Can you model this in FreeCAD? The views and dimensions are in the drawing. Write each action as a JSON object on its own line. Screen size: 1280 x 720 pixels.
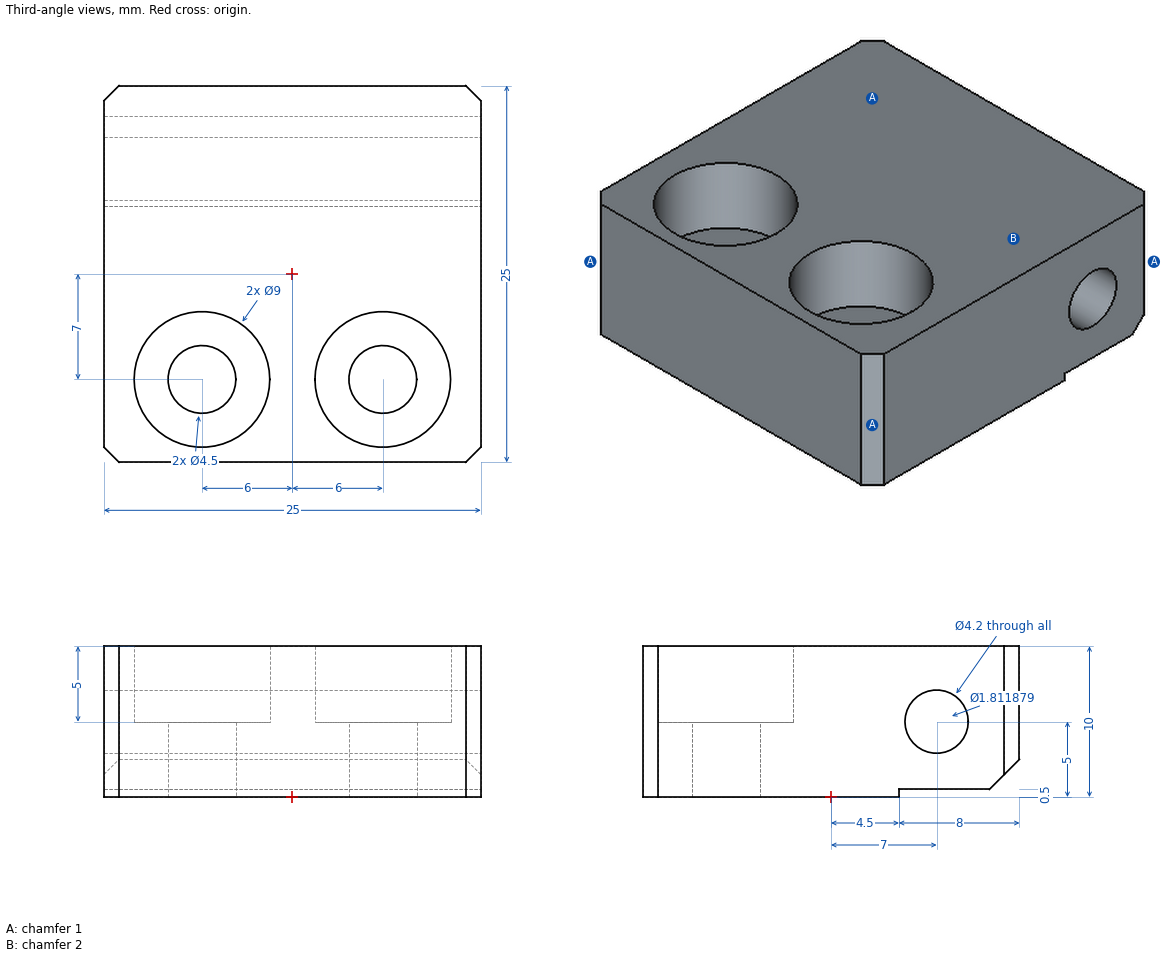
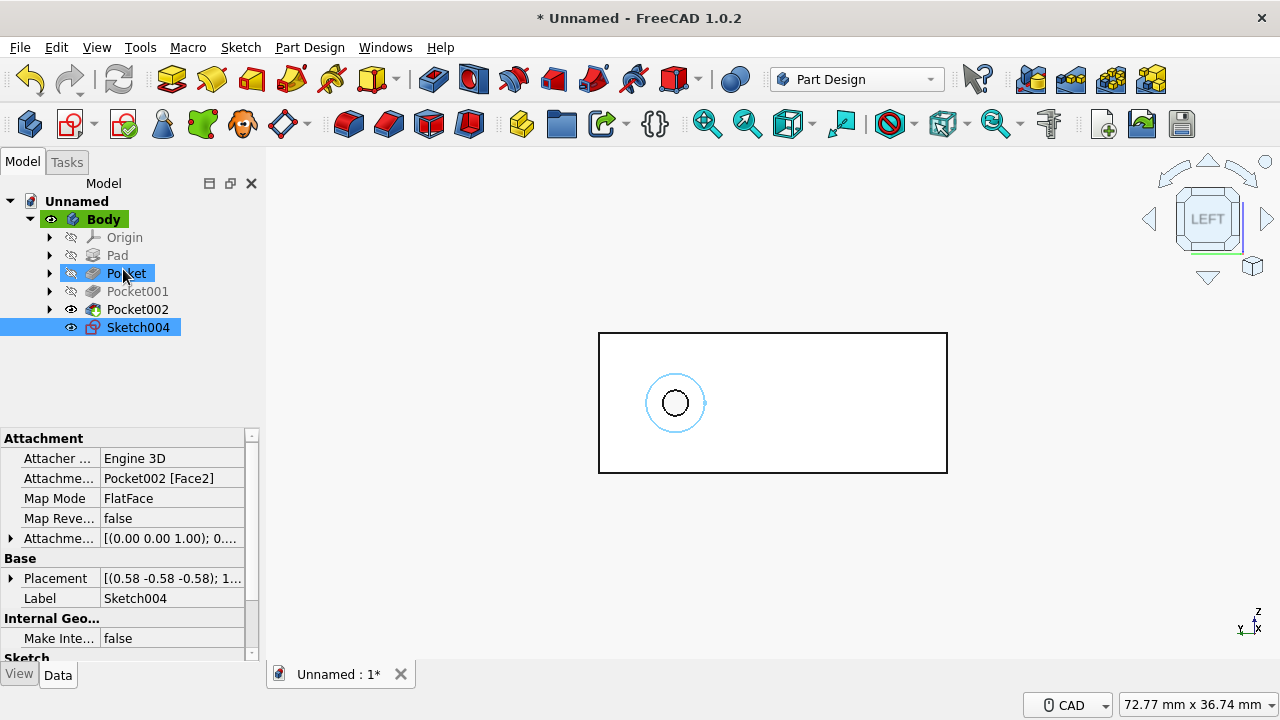
{"action": "left_click", "coordinate": [474, 80]}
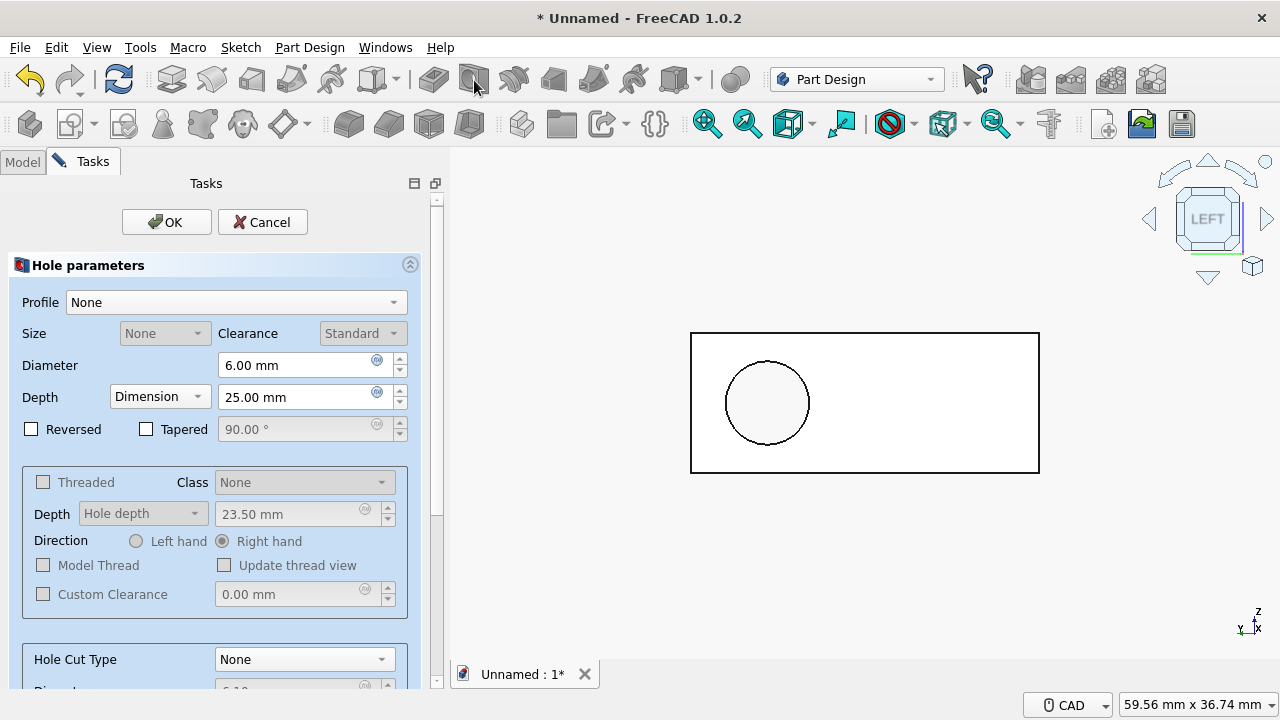
{"action": "triple_click", "coordinate": [305, 365]}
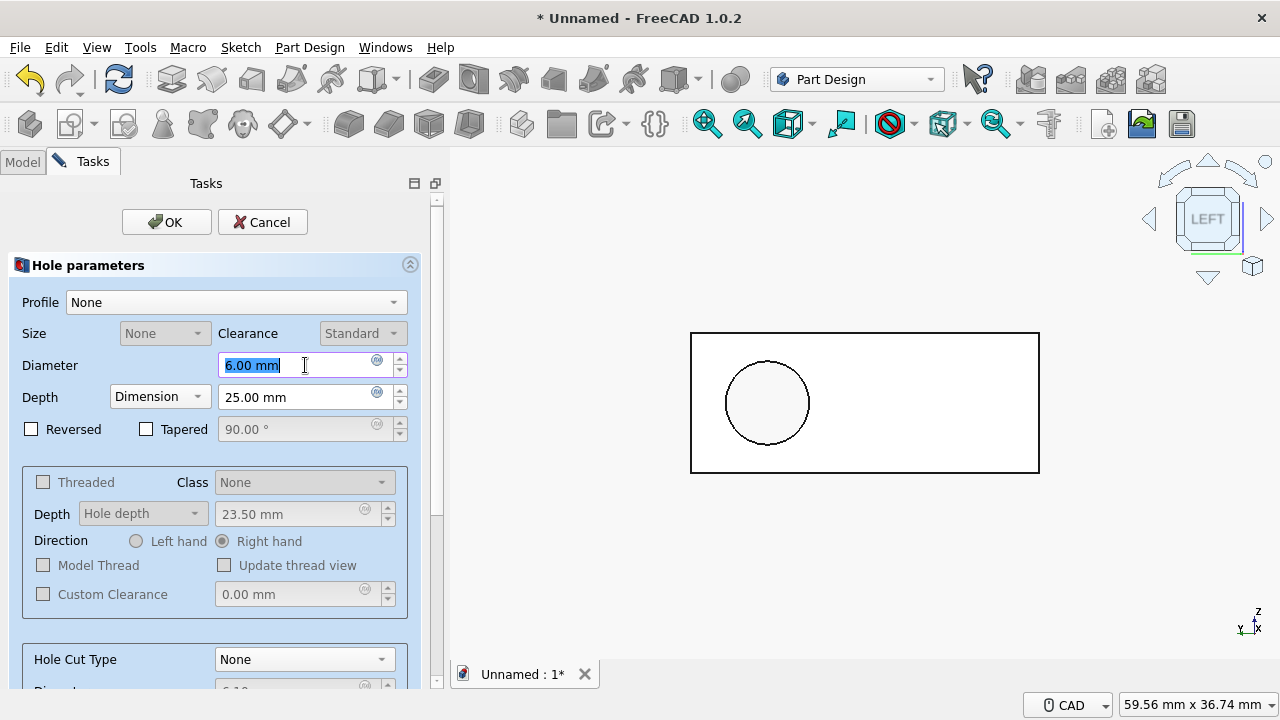
{"action": "type", "text": "4.2"}
{"action": "key", "text": "Tab"}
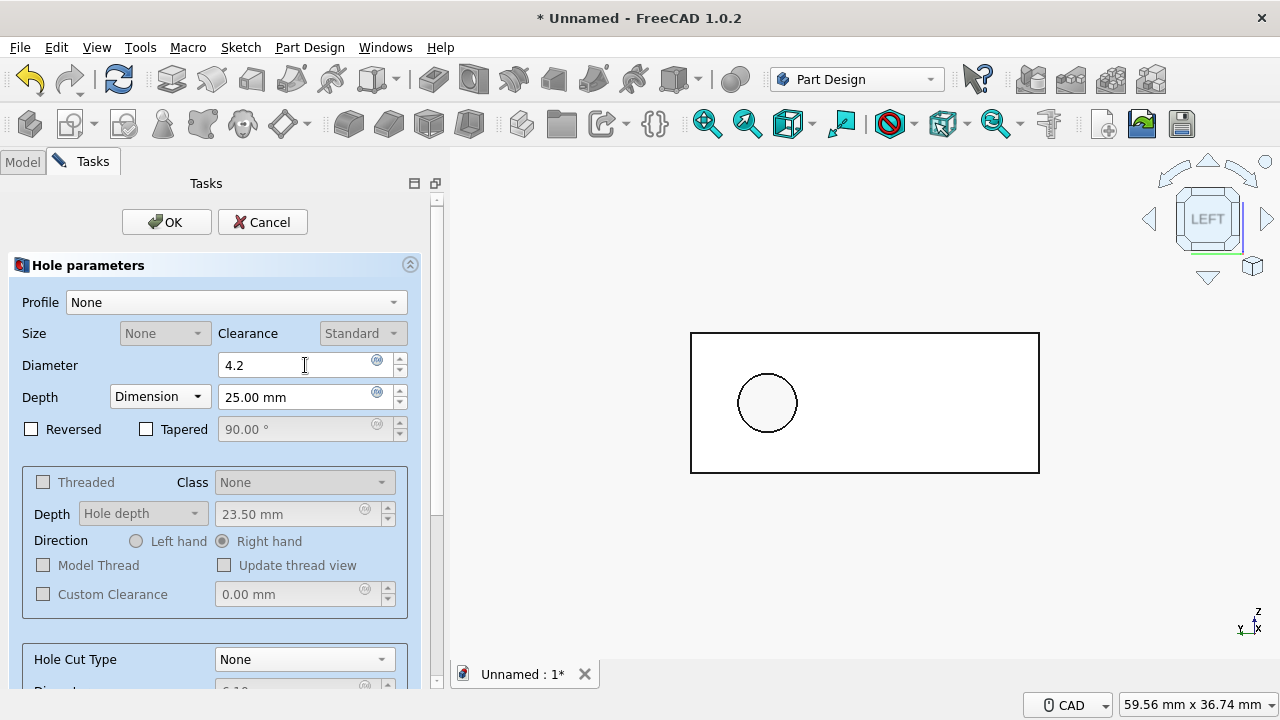
{"action": "left_click", "coordinate": [161, 396]}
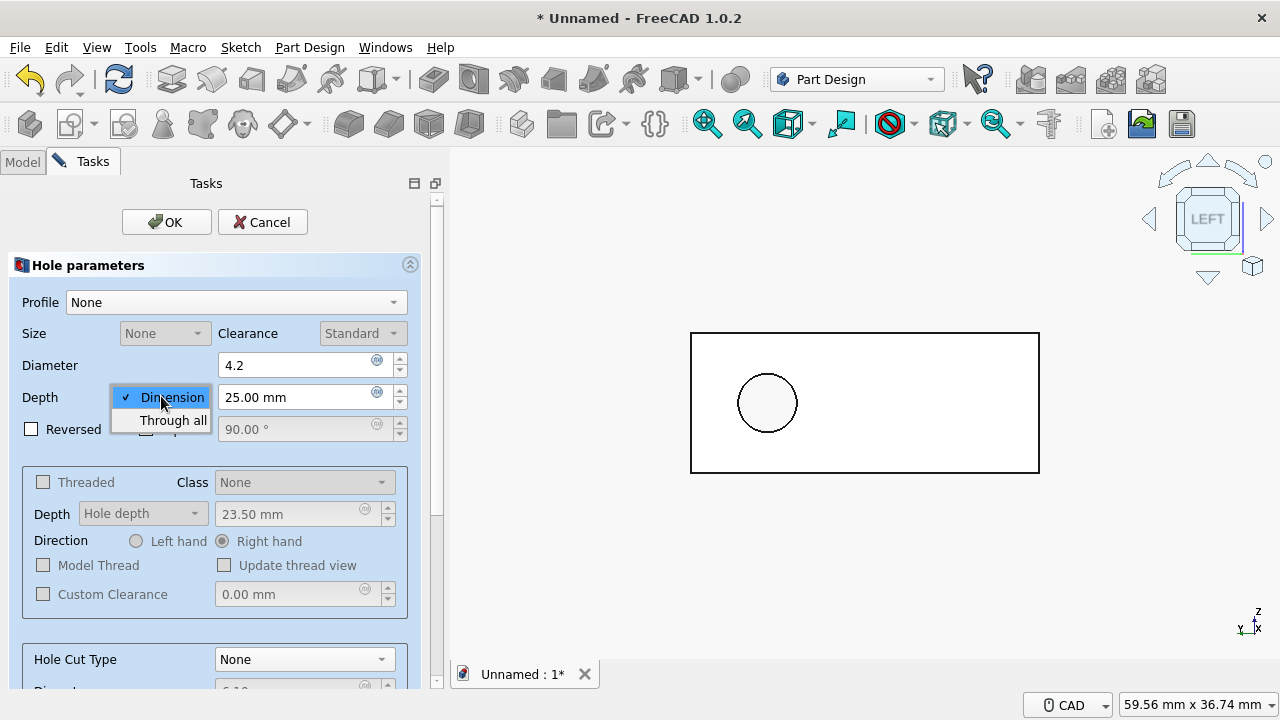
{"action": "left_click", "coordinate": [160, 420]}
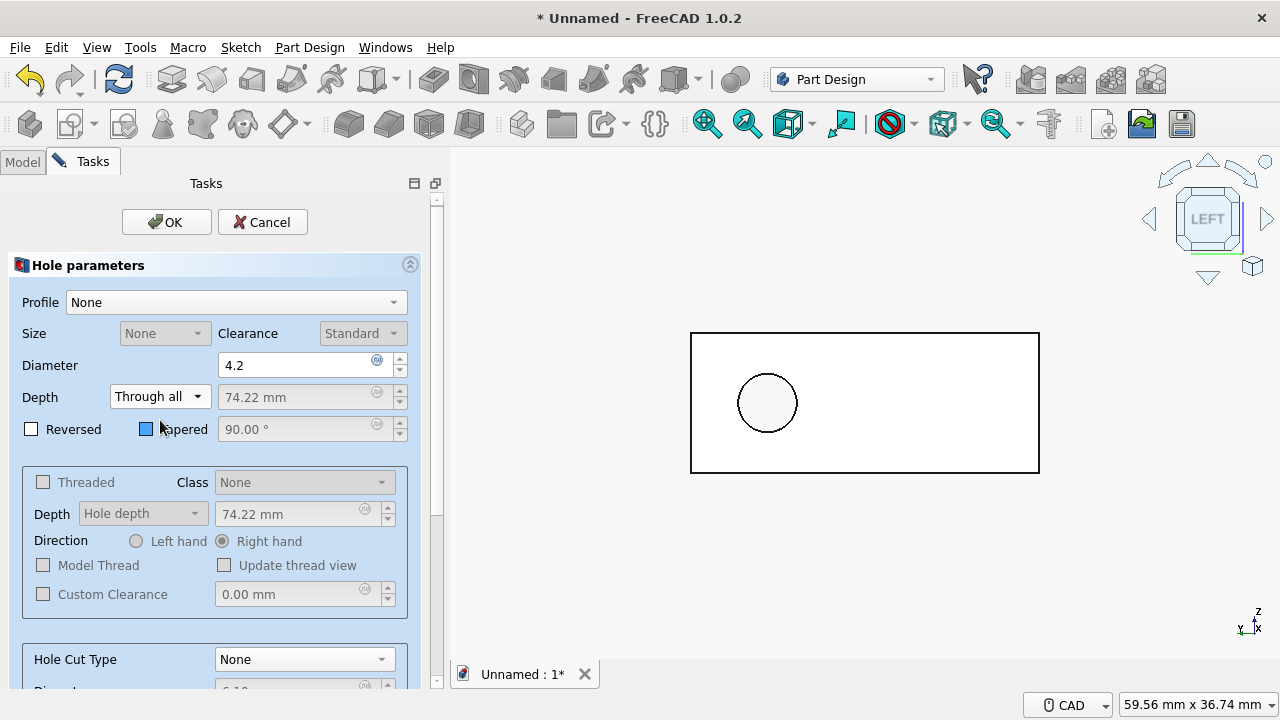
{"action": "left_click", "coordinate": [167, 222]}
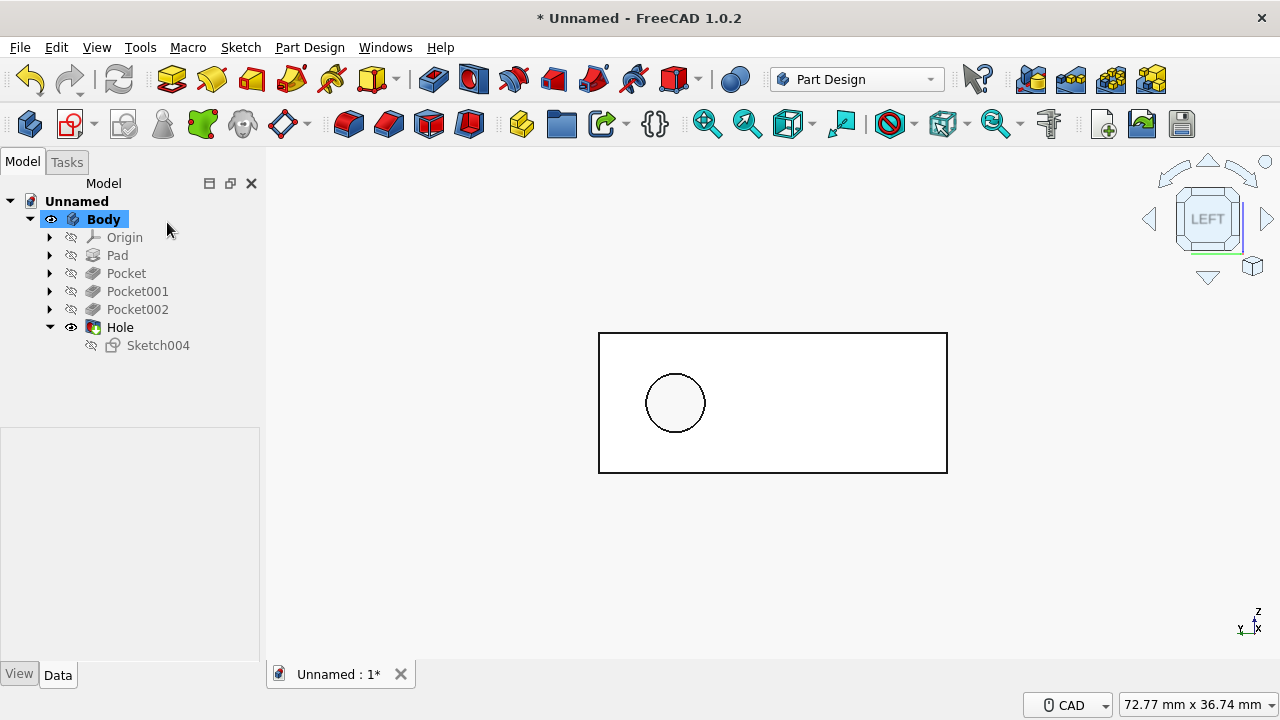
{"action": "key", "text": "v f"}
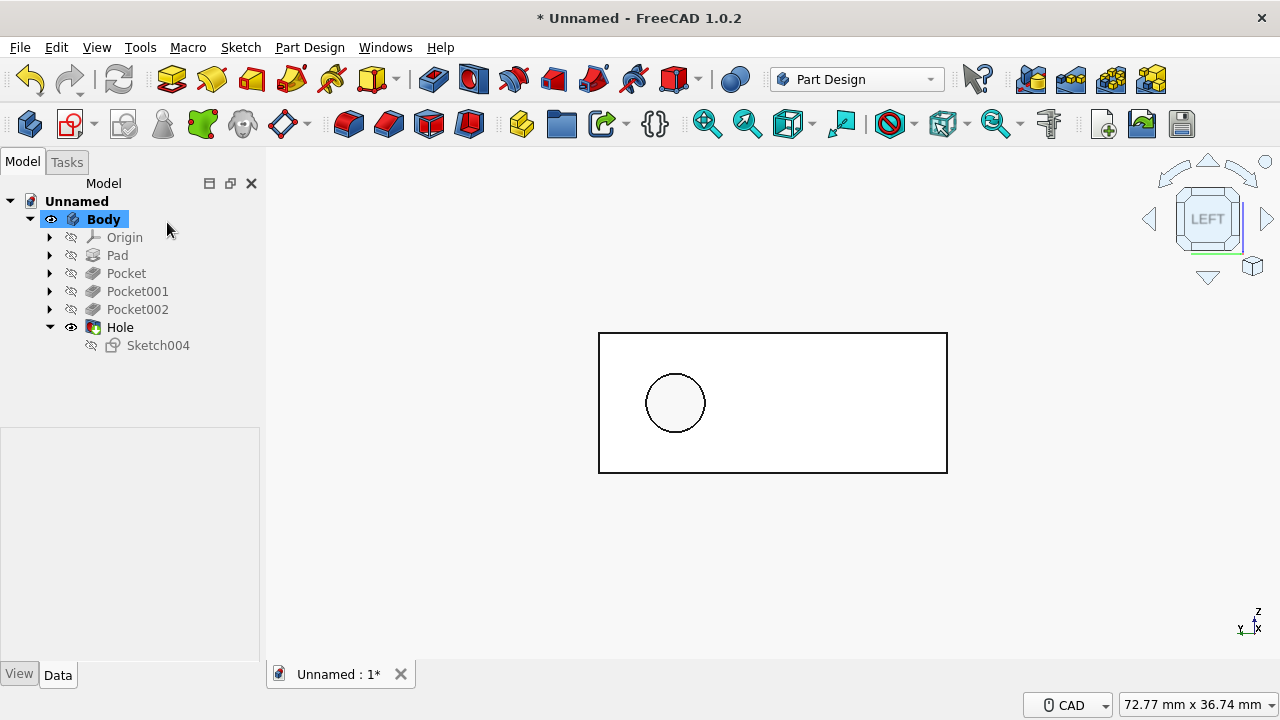
{"action": "left_click", "coordinate": [947, 402]}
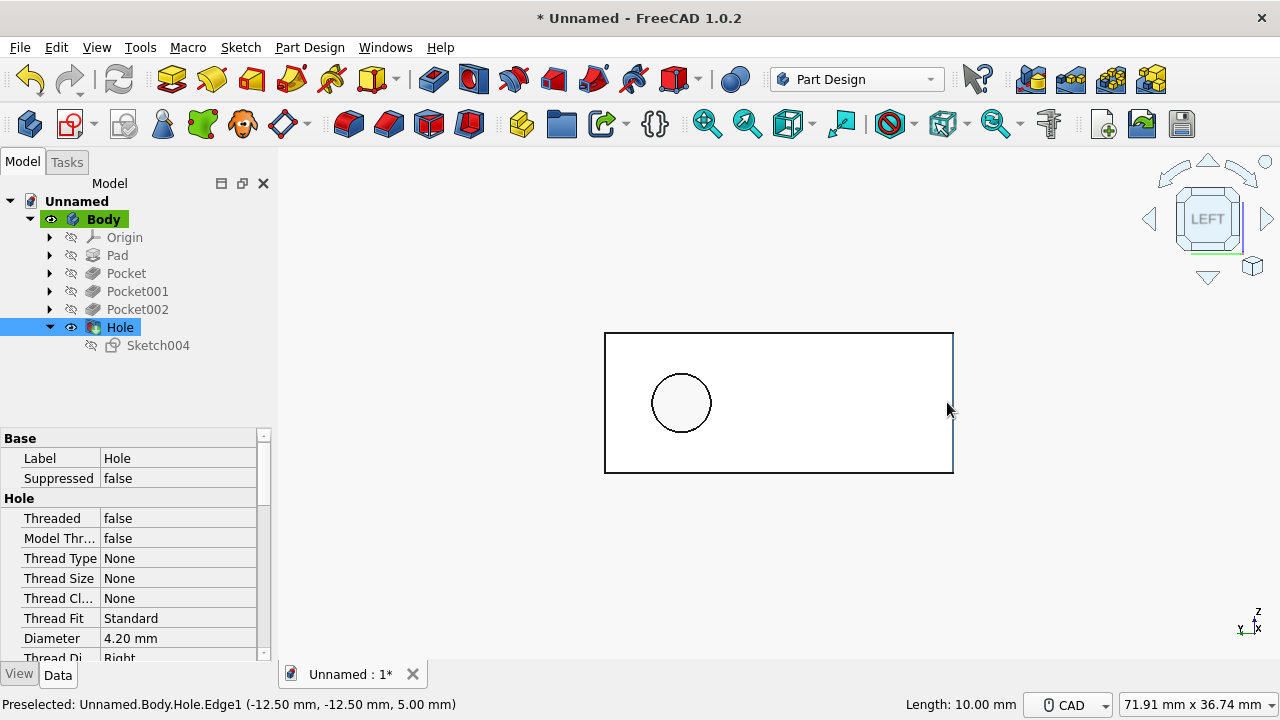
{"action": "left_click", "coordinate": [605, 402], "text": "ctrl"}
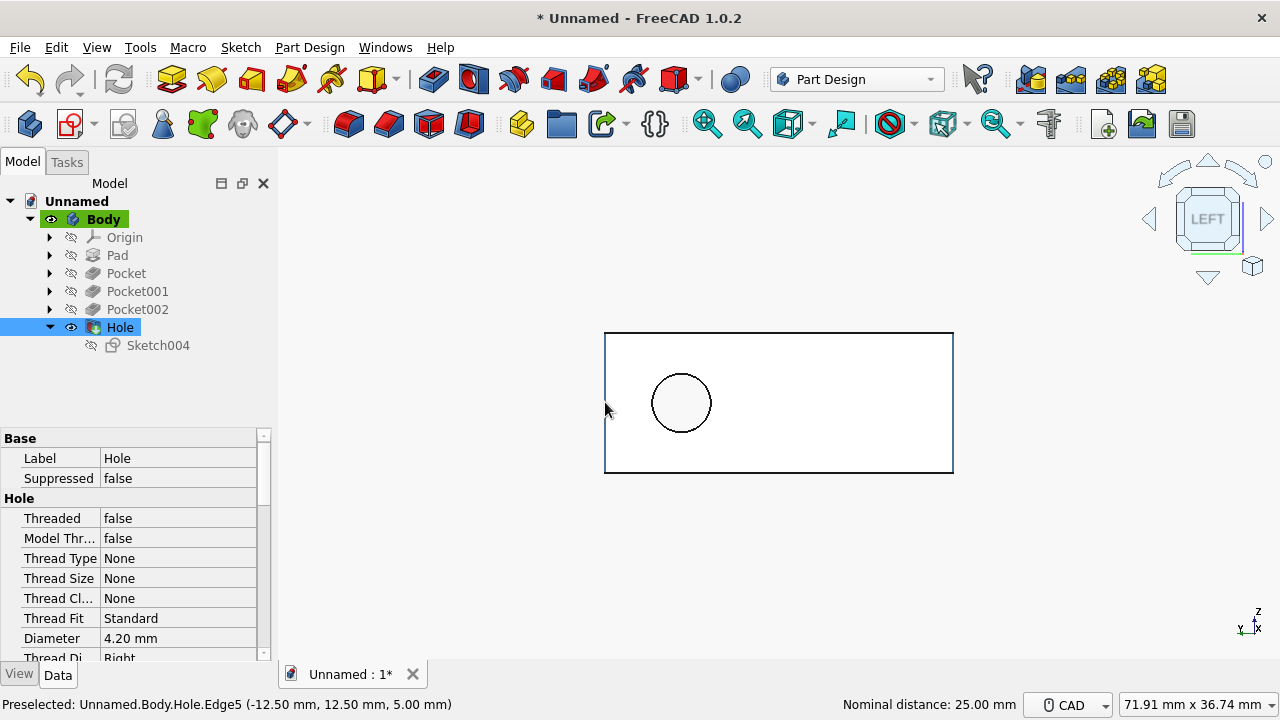
{"action": "key", "text": "0"}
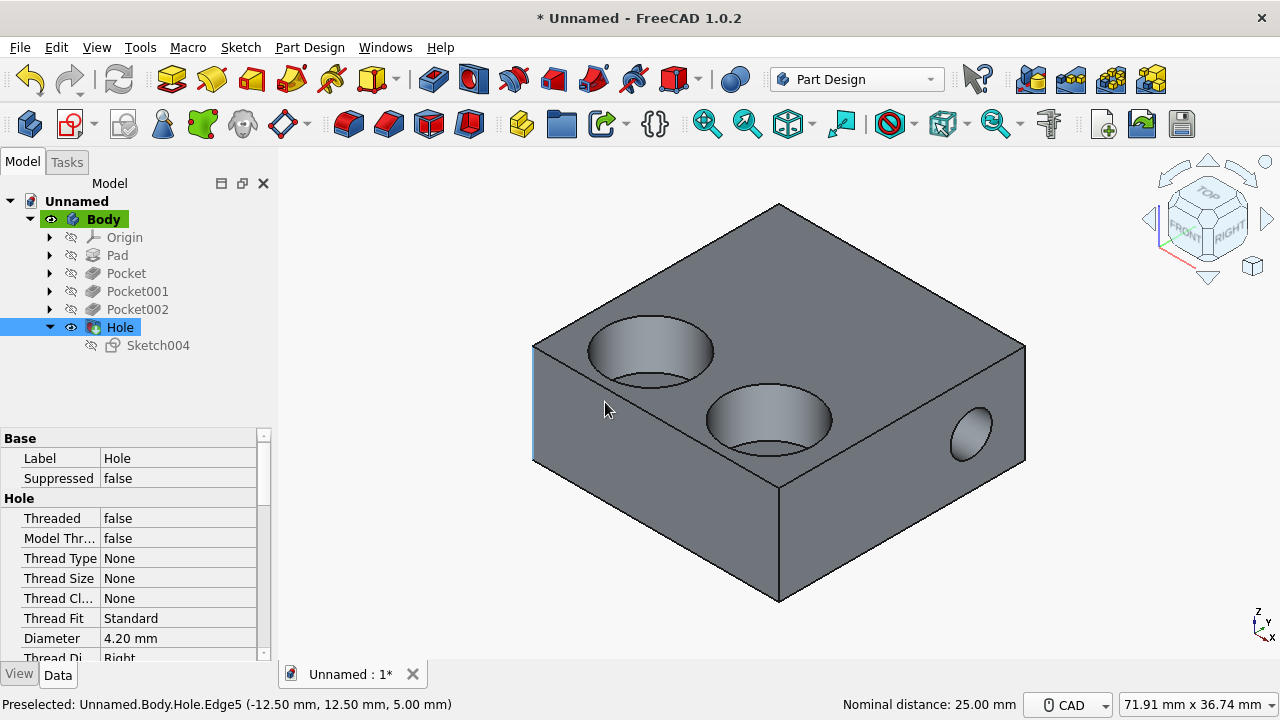
{"action": "left_click", "coordinate": [779, 544], "text": "ctrl"}